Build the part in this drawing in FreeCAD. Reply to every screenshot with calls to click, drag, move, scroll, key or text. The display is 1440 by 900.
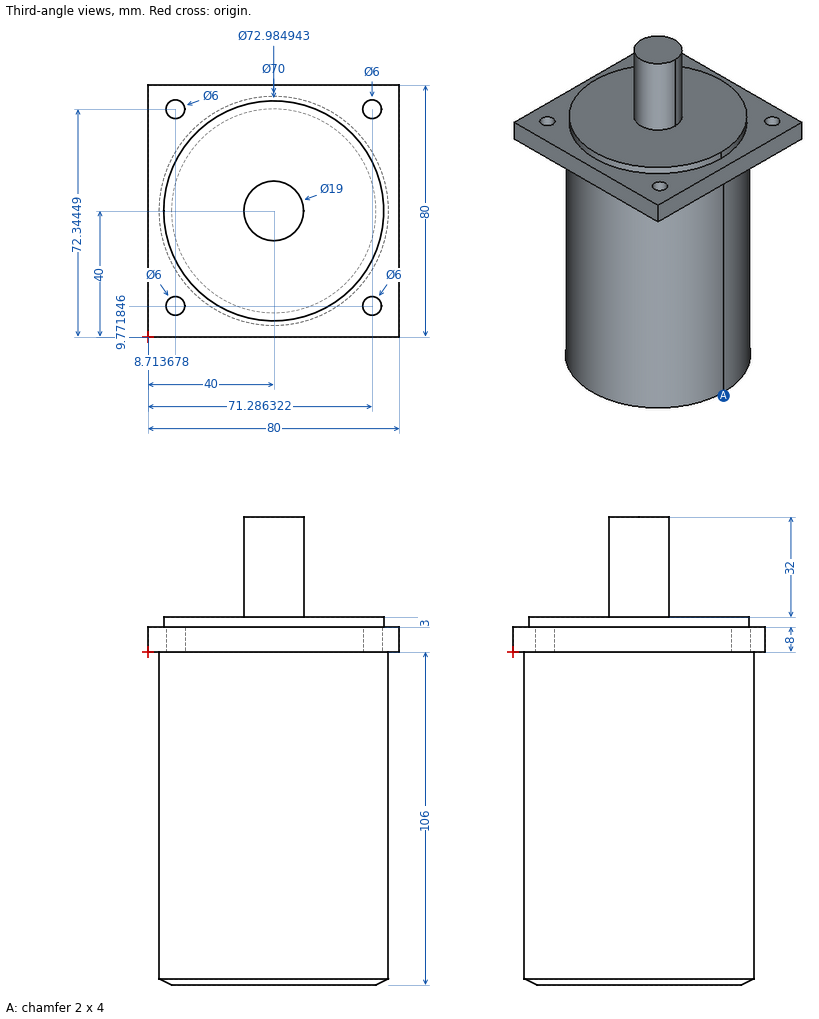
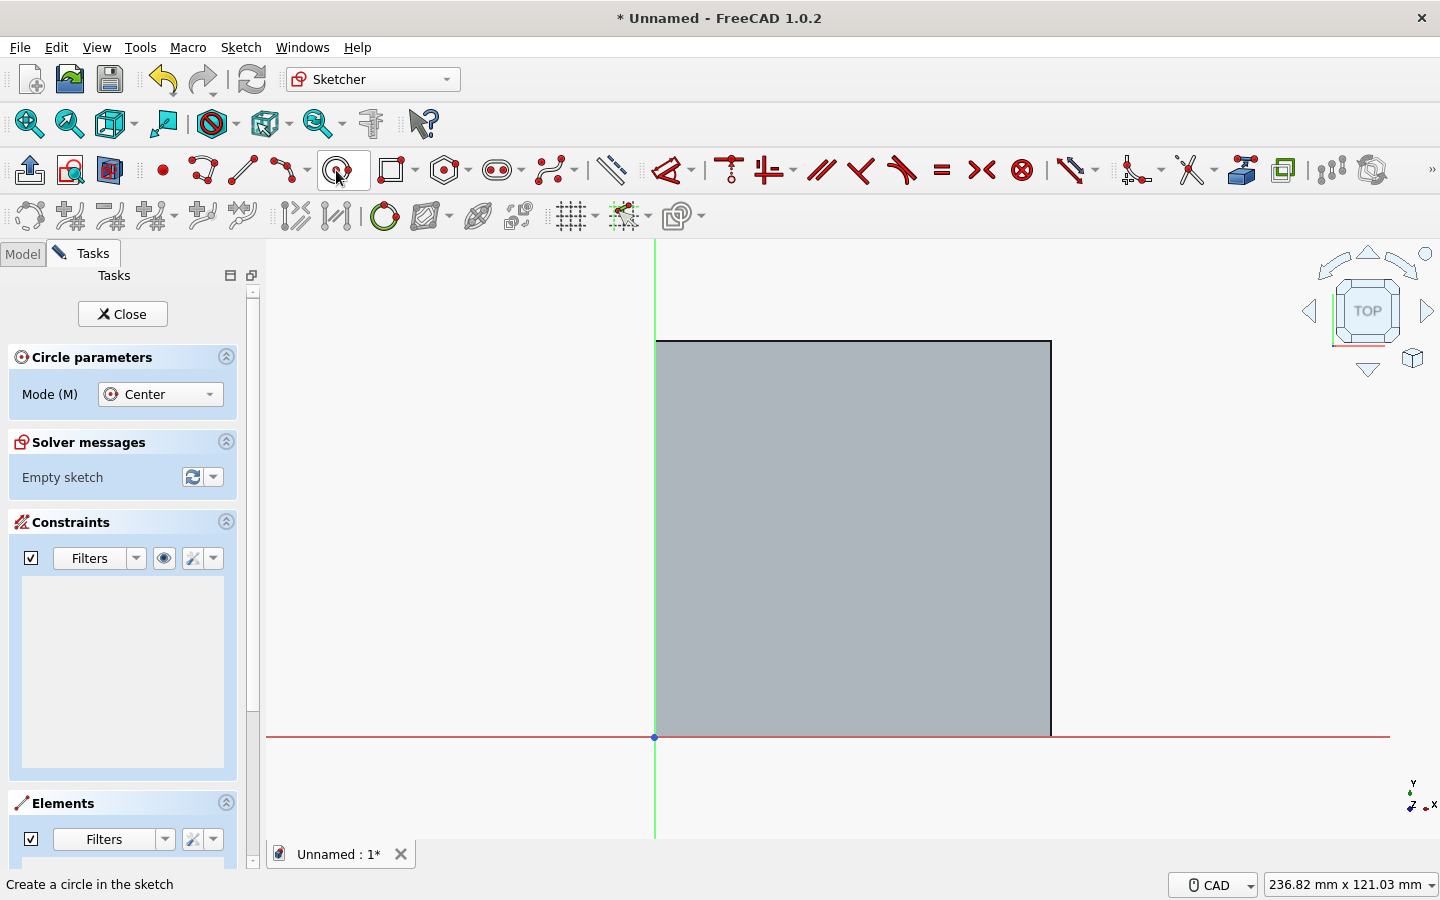
click(853, 539)
move(981, 411)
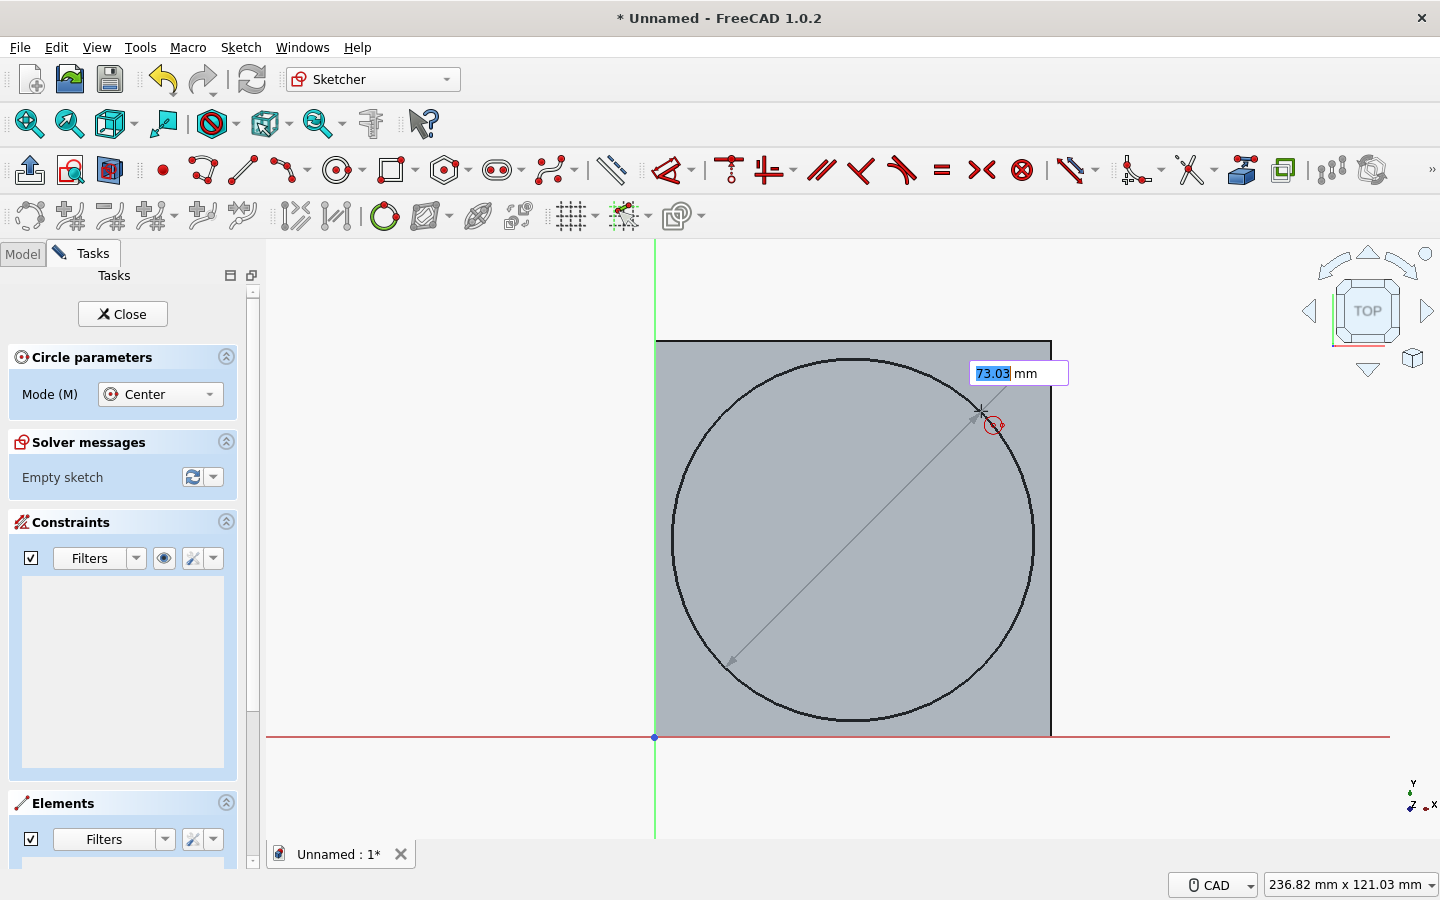
text(72.984943)
key(Return)
key(Escape)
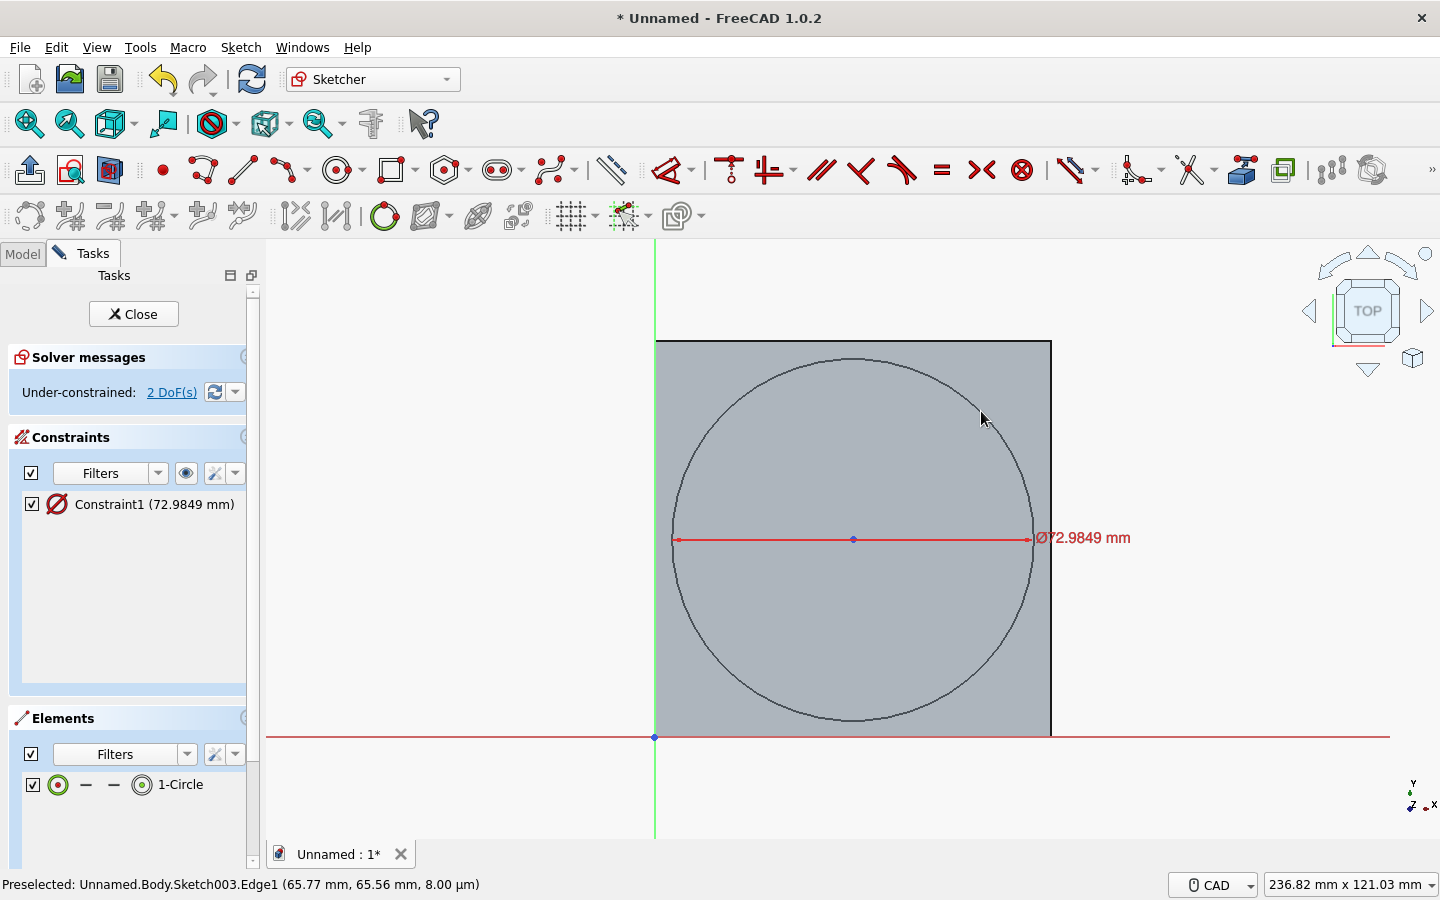
click(666, 170)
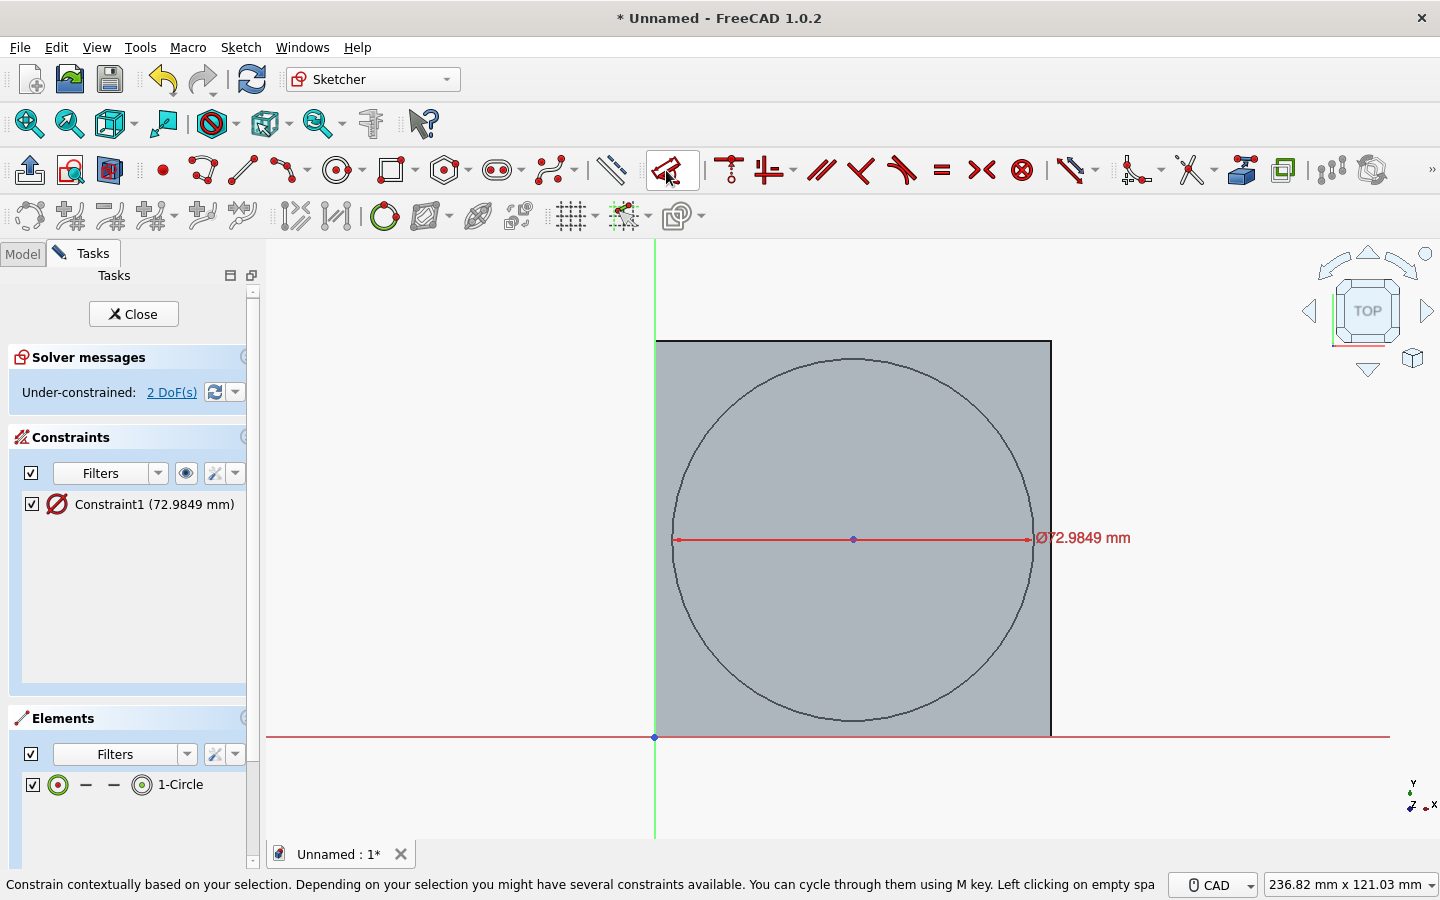
click(853, 540)
click(754, 771)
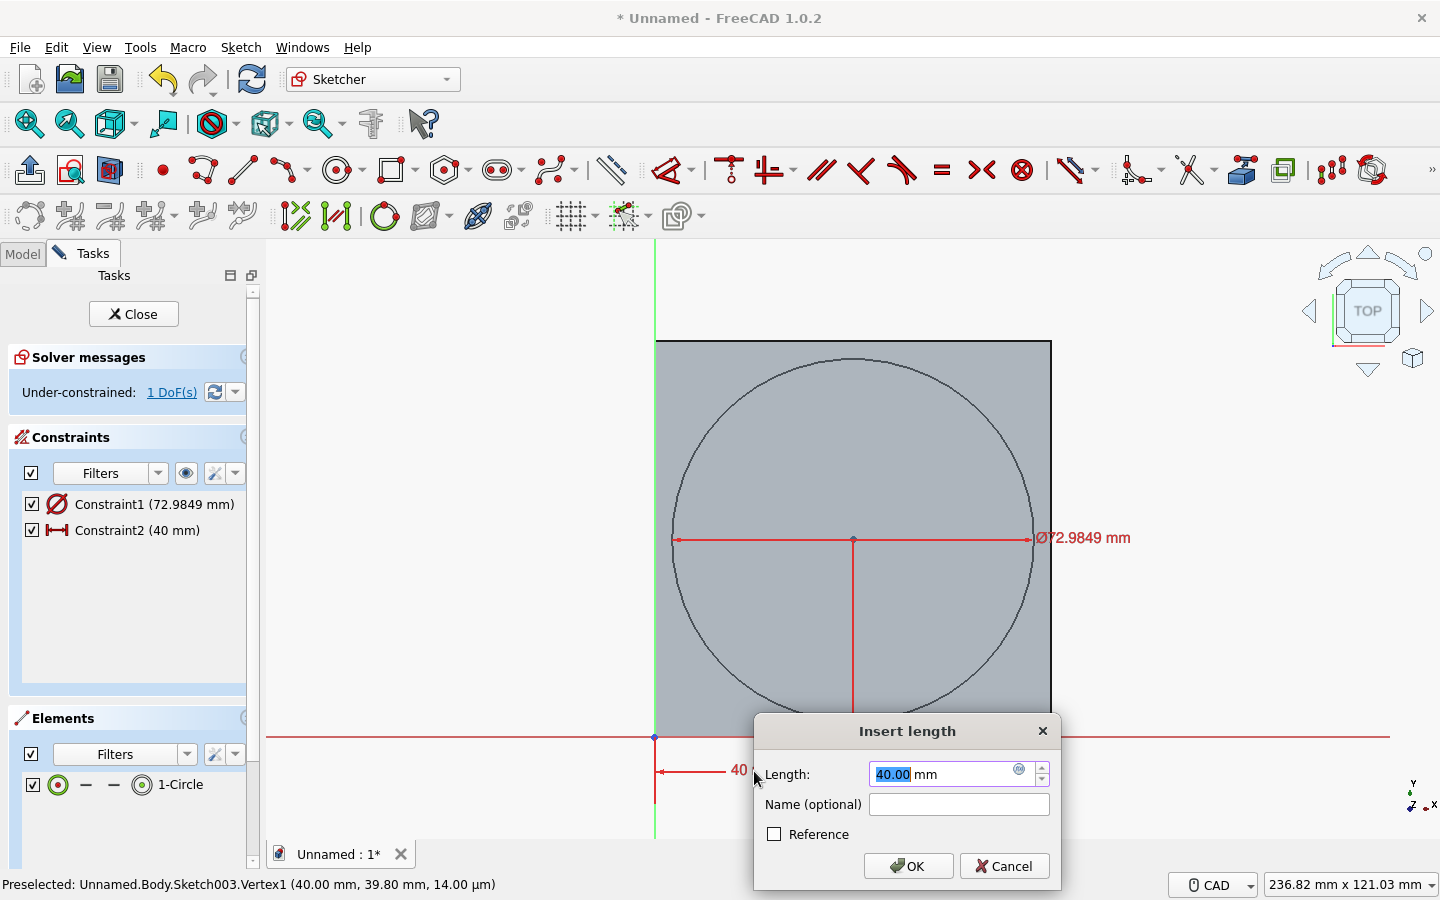
text(40)
key(Return)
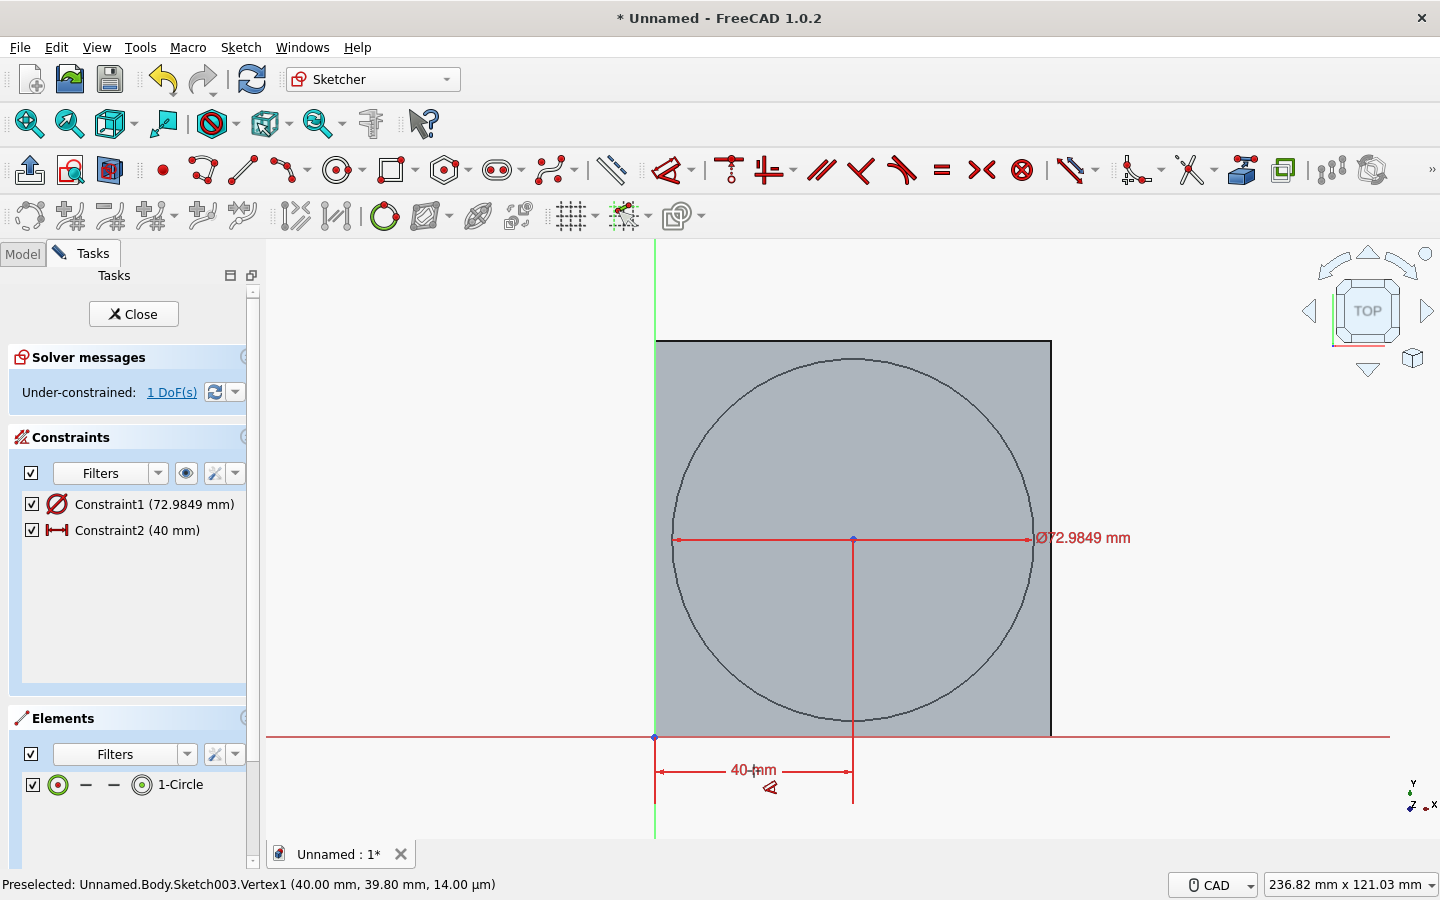
click(853, 540)
click(621, 639)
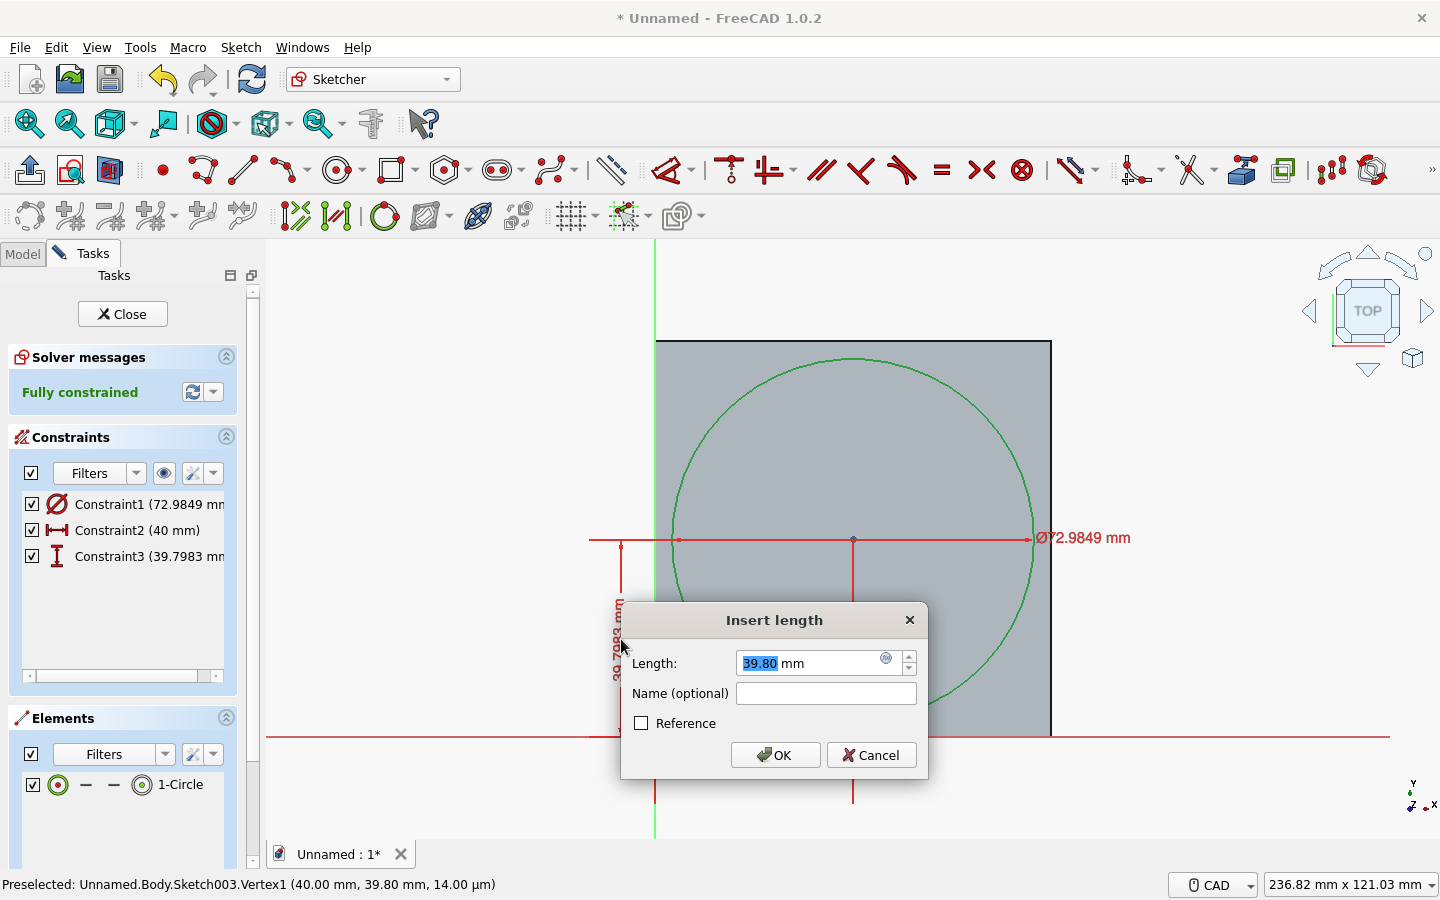
text(40)
key(Return)
key(Escape)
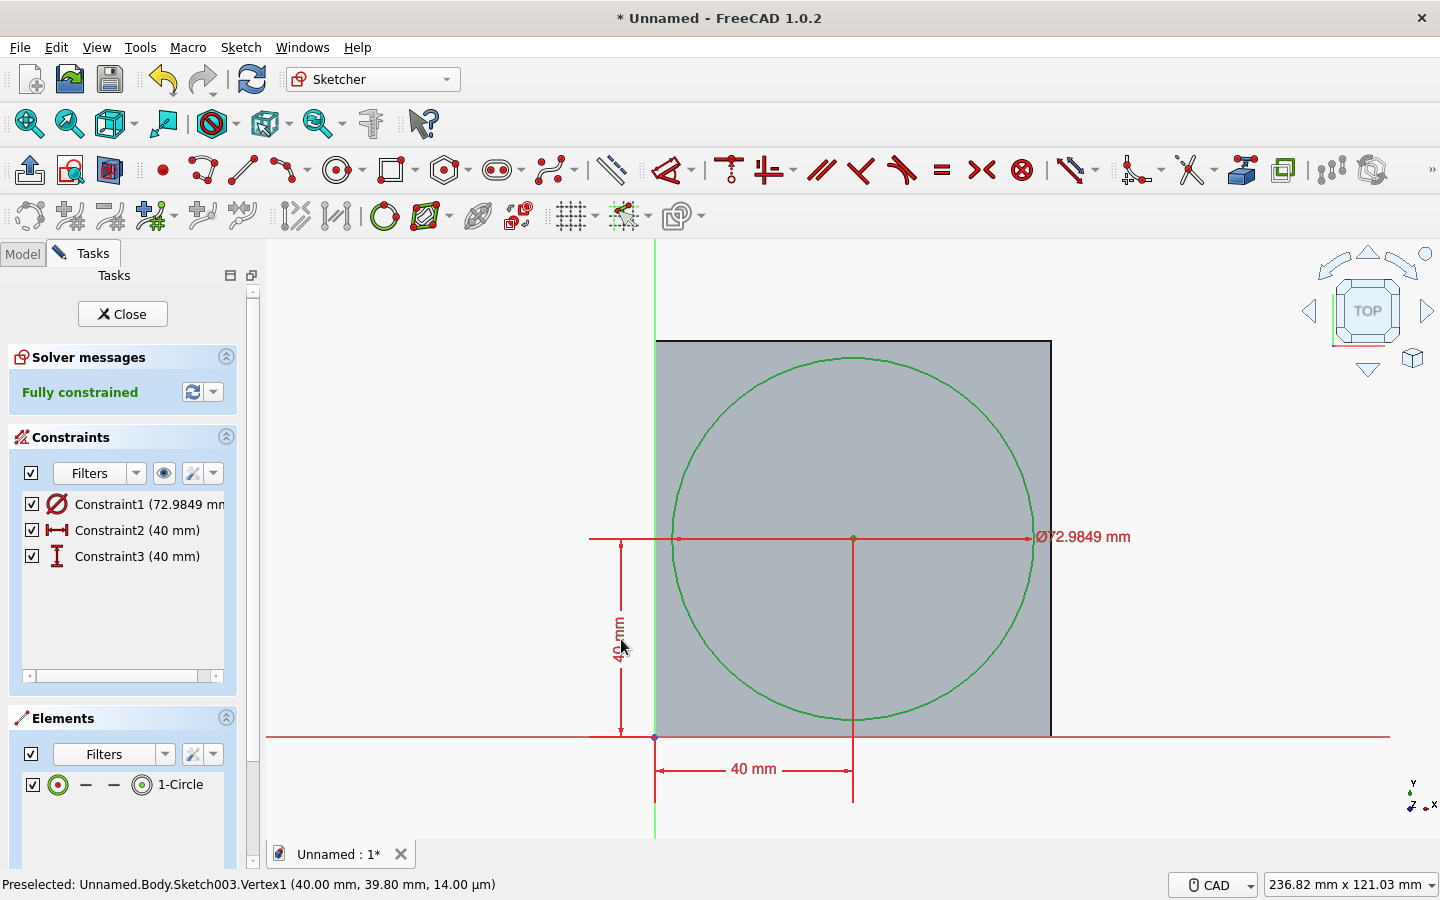
click(123, 314)